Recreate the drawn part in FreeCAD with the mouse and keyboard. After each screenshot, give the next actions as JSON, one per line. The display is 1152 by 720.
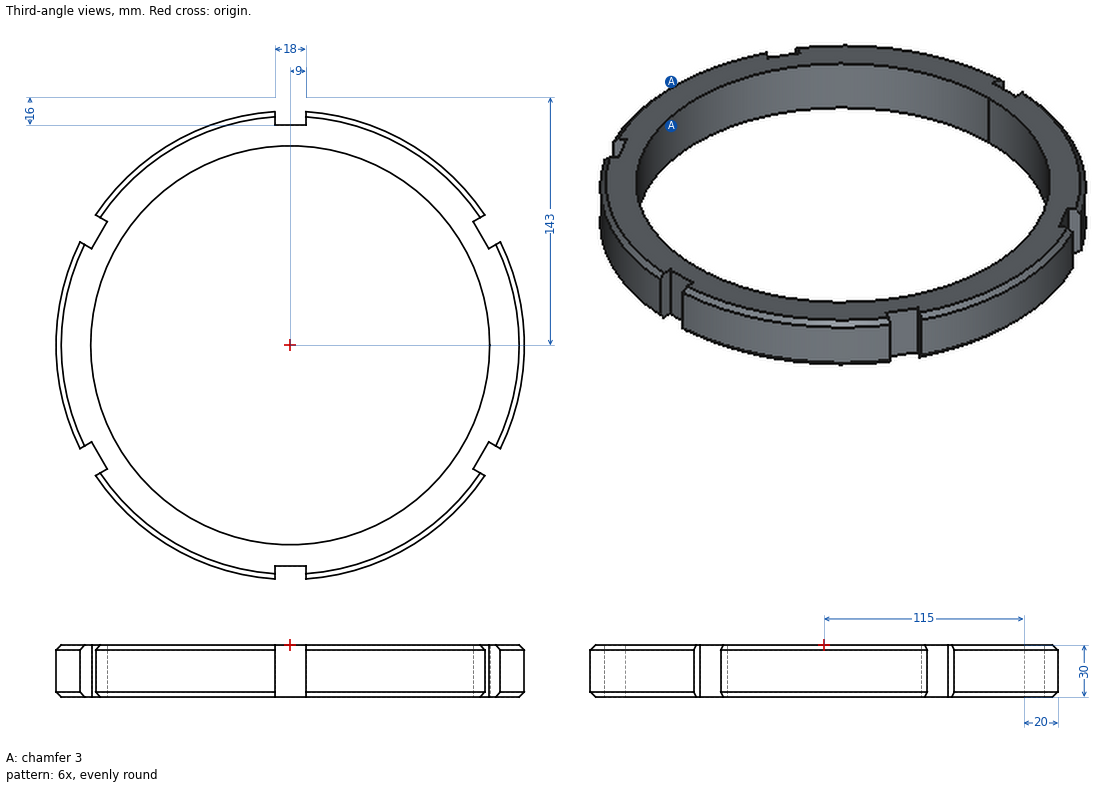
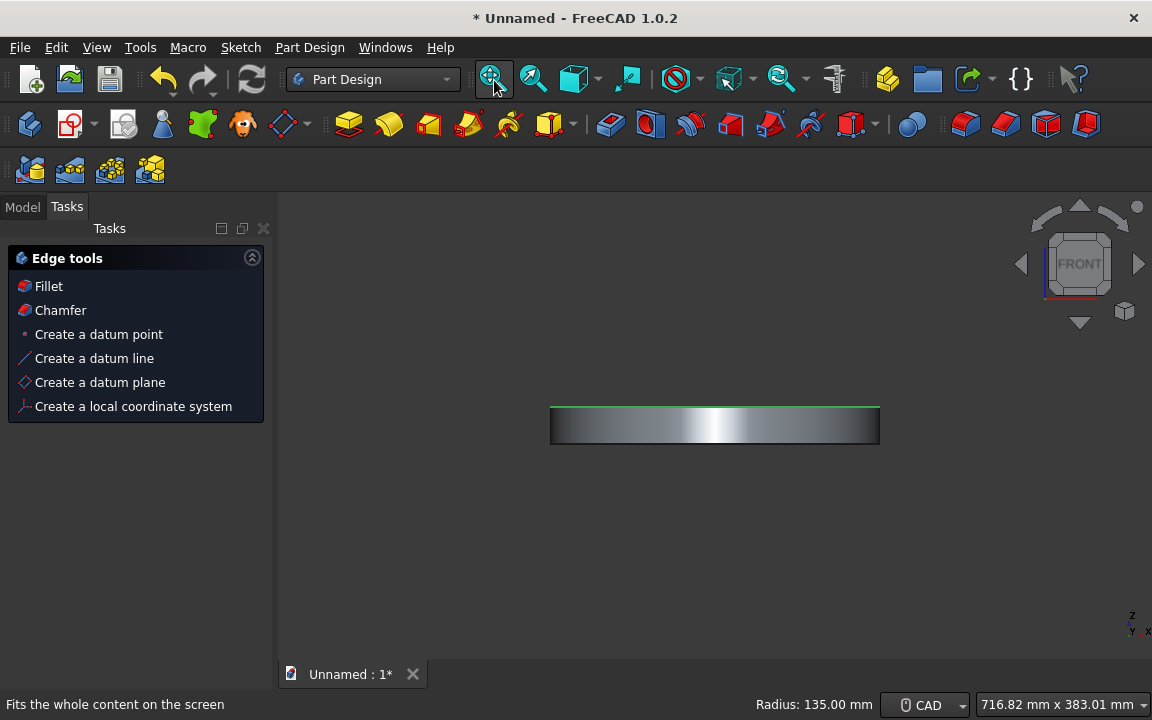
{"action": "left_click", "coordinate": [715, 443], "text": "ctrl"}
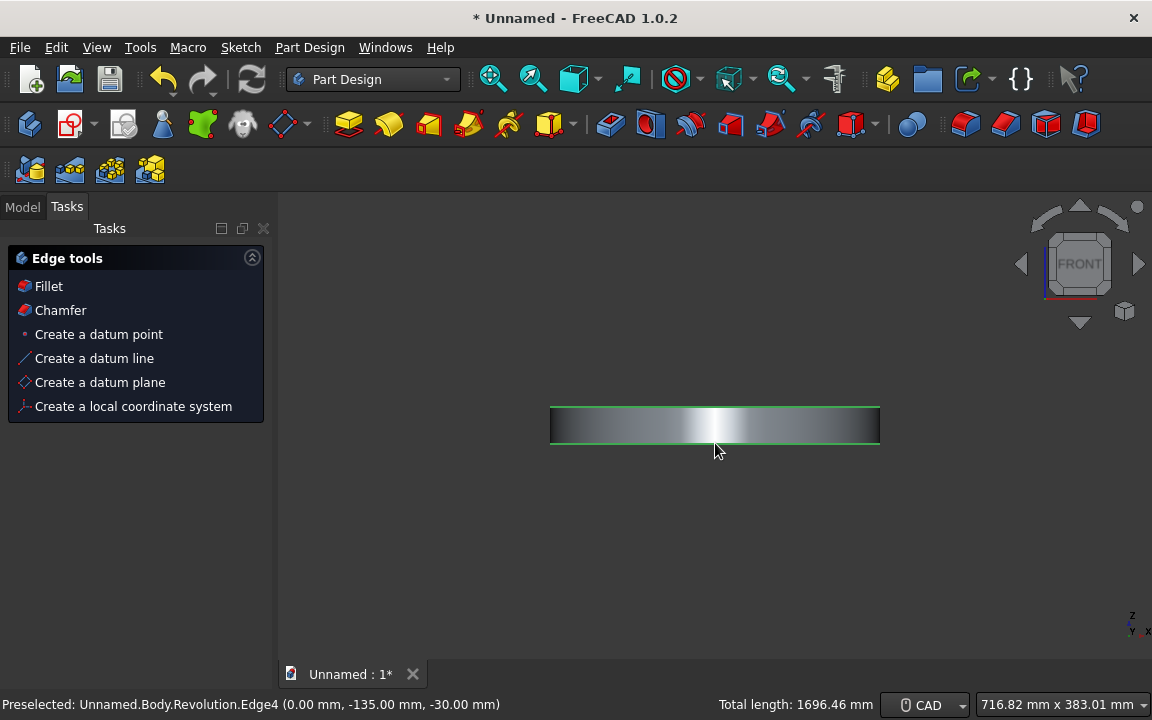
{"action": "left_click", "coordinate": [1006, 124]}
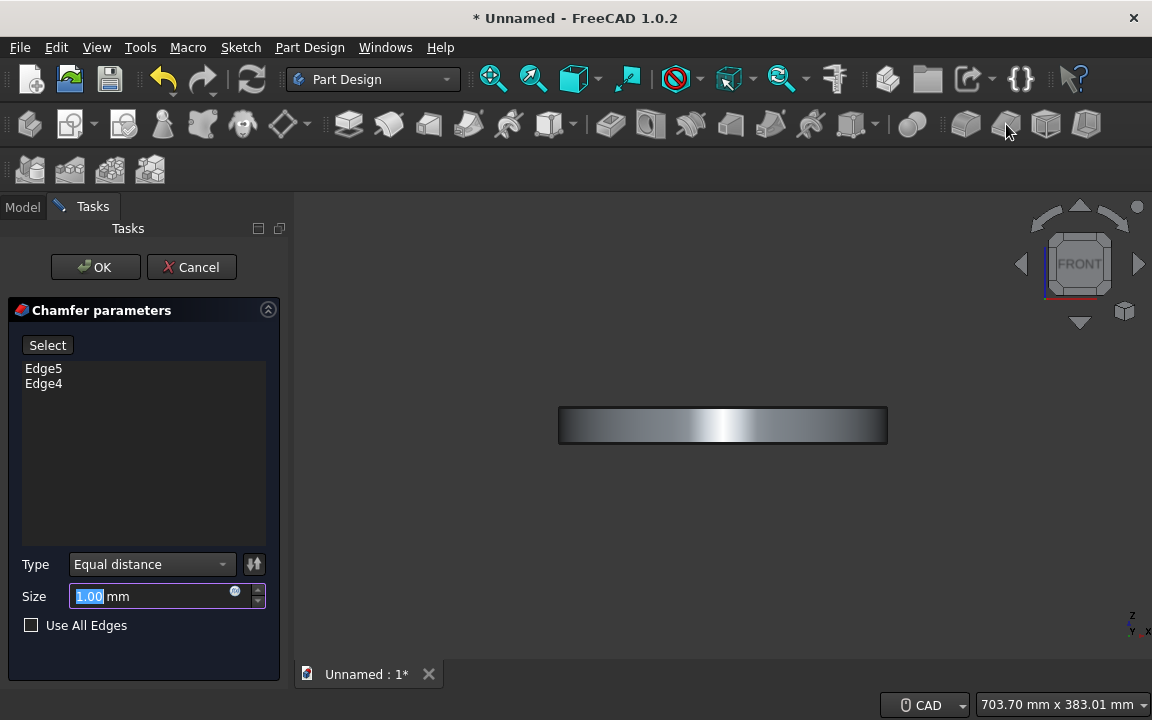
{"action": "type", "text": "3"}
{"action": "key", "text": "Tab"}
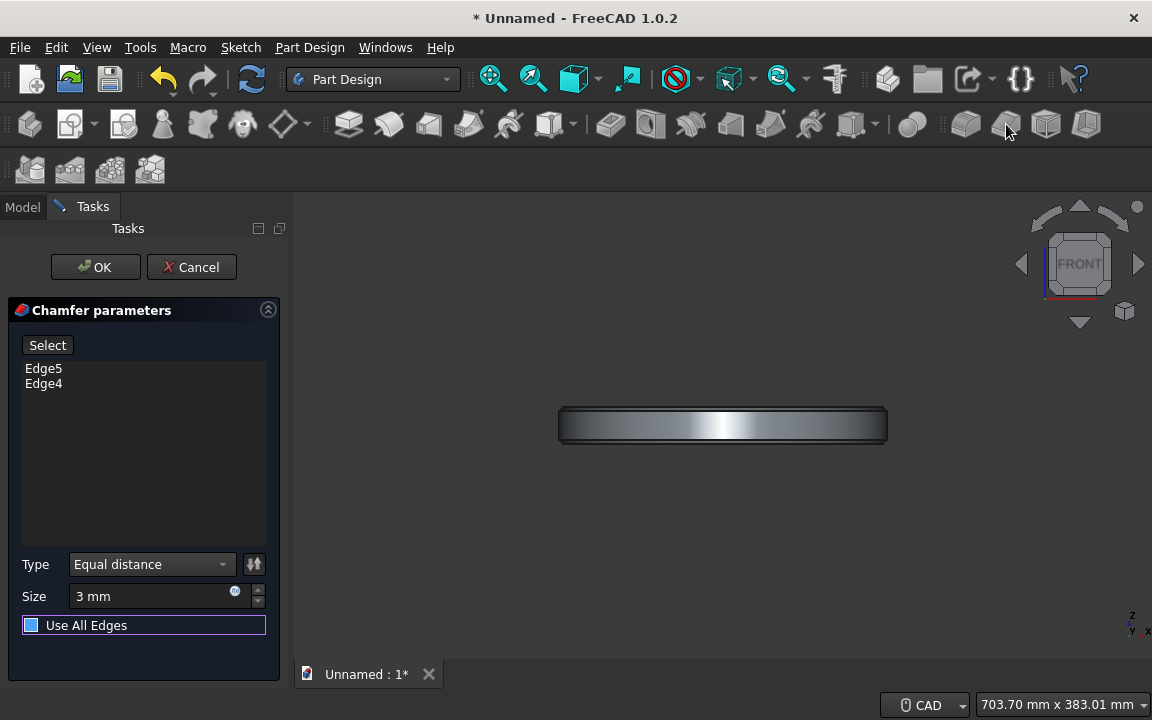
{"action": "left_click", "coordinate": [96, 267]}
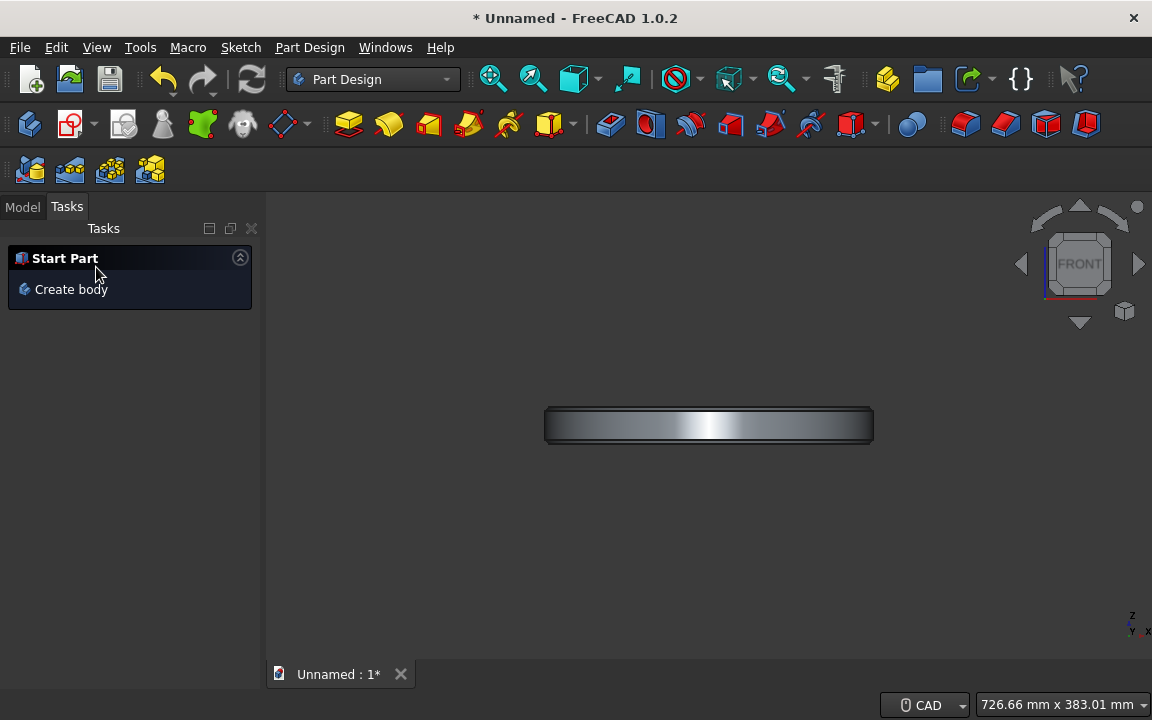
{"action": "left_click", "coordinate": [494, 80]}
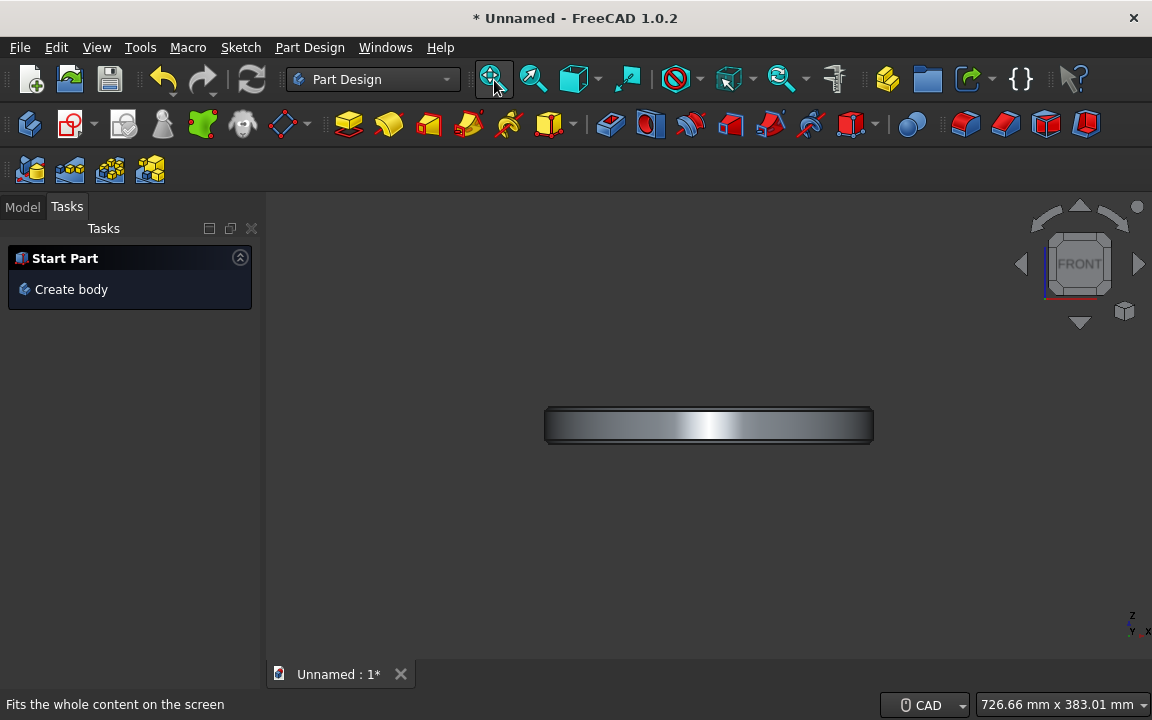
{"action": "key", "text": "0"}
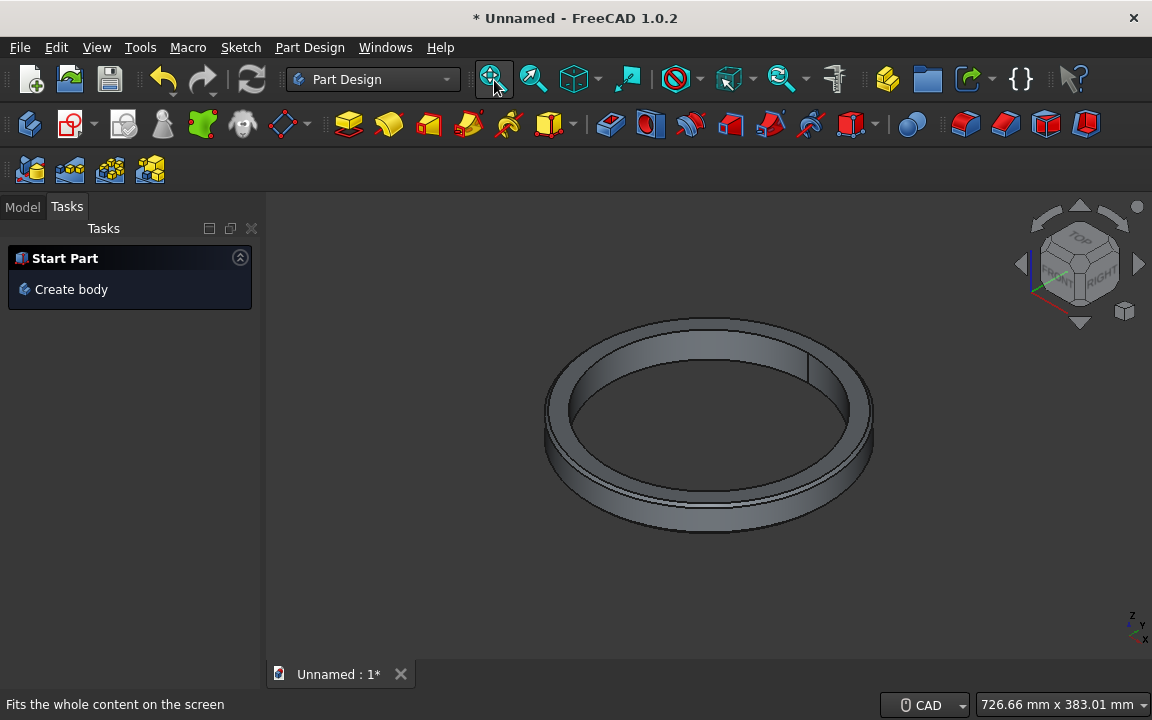
{"action": "left_click", "coordinate": [579, 447]}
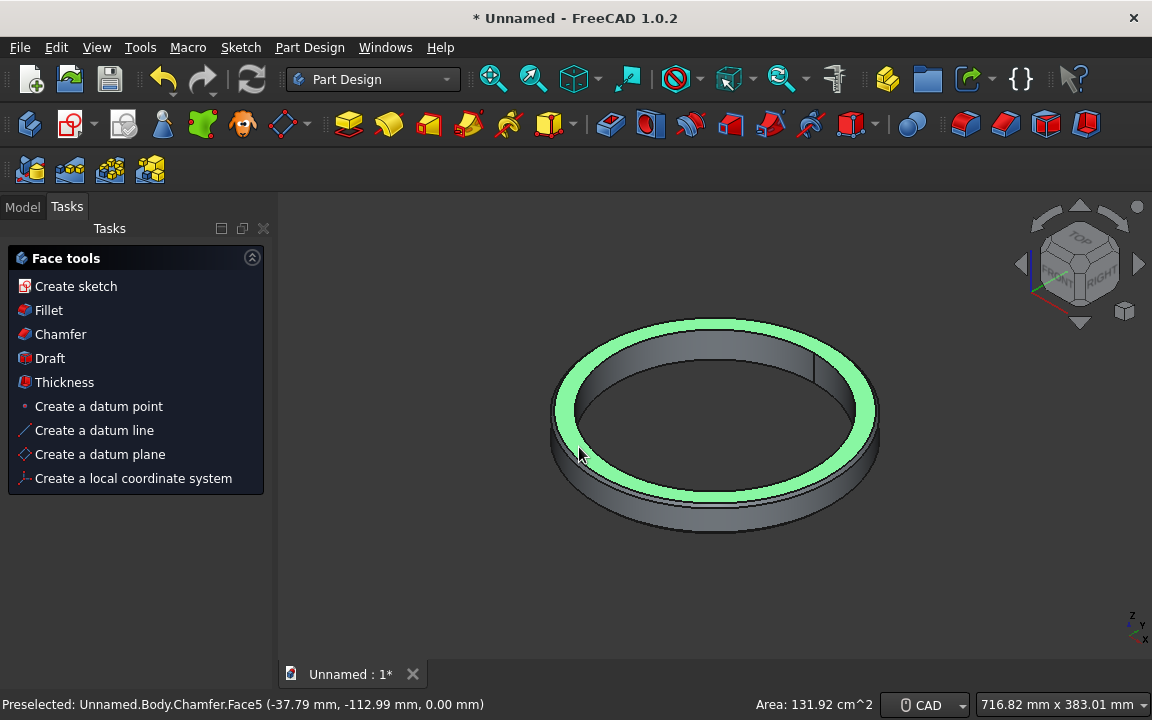
{"action": "left_click", "coordinate": [70, 124]}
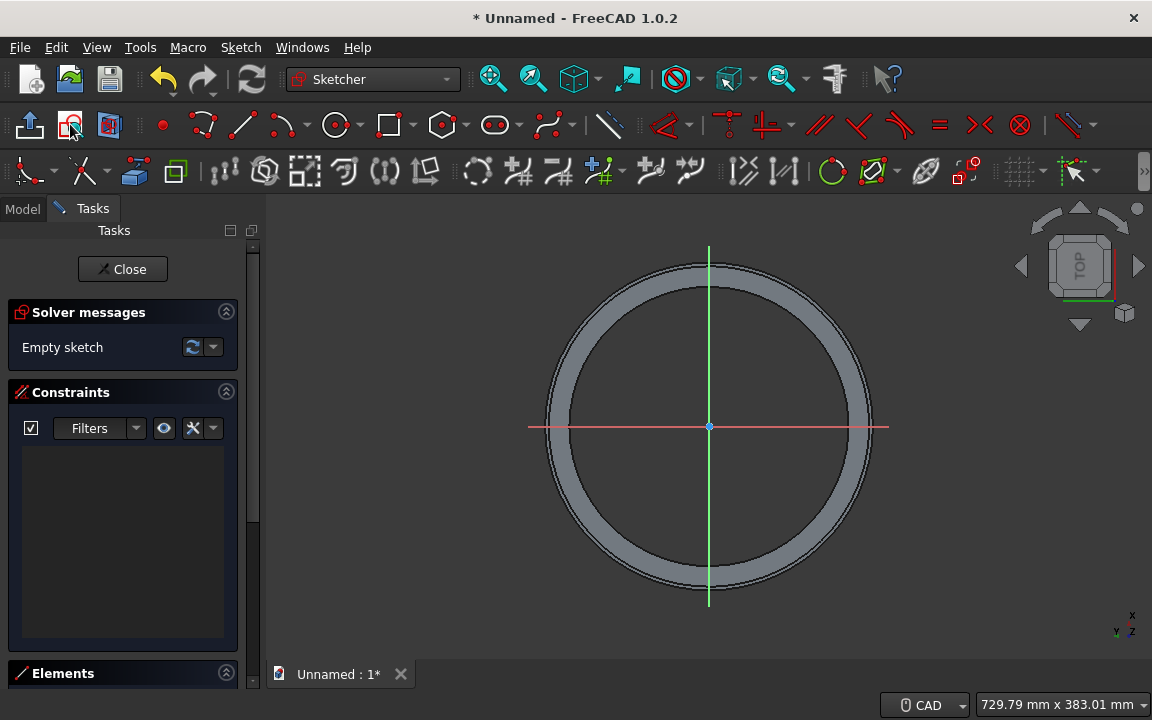
{"action": "scroll", "coordinate": [537, 426], "scroll_direction": "up", "scroll_amount": 13}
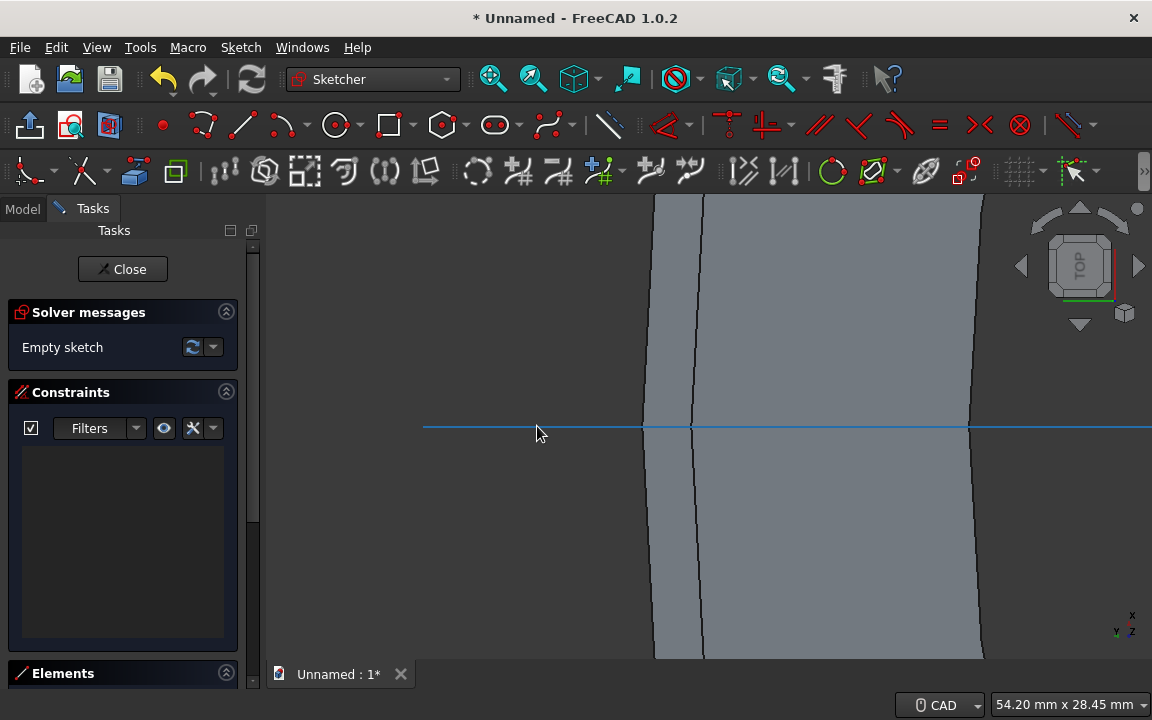
{"action": "left_click", "coordinate": [390, 126]}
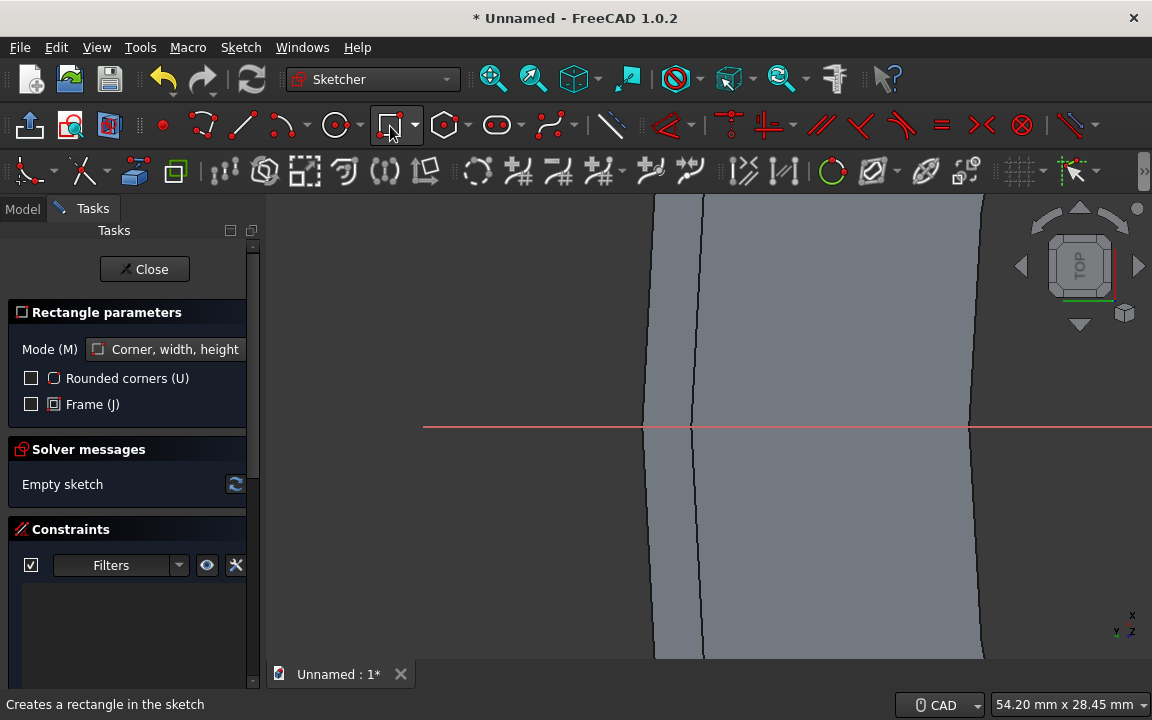
{"action": "left_click", "coordinate": [512, 279]}
{"action": "left_click", "coordinate": [773, 574]}
{"action": "key", "text": "Escape"}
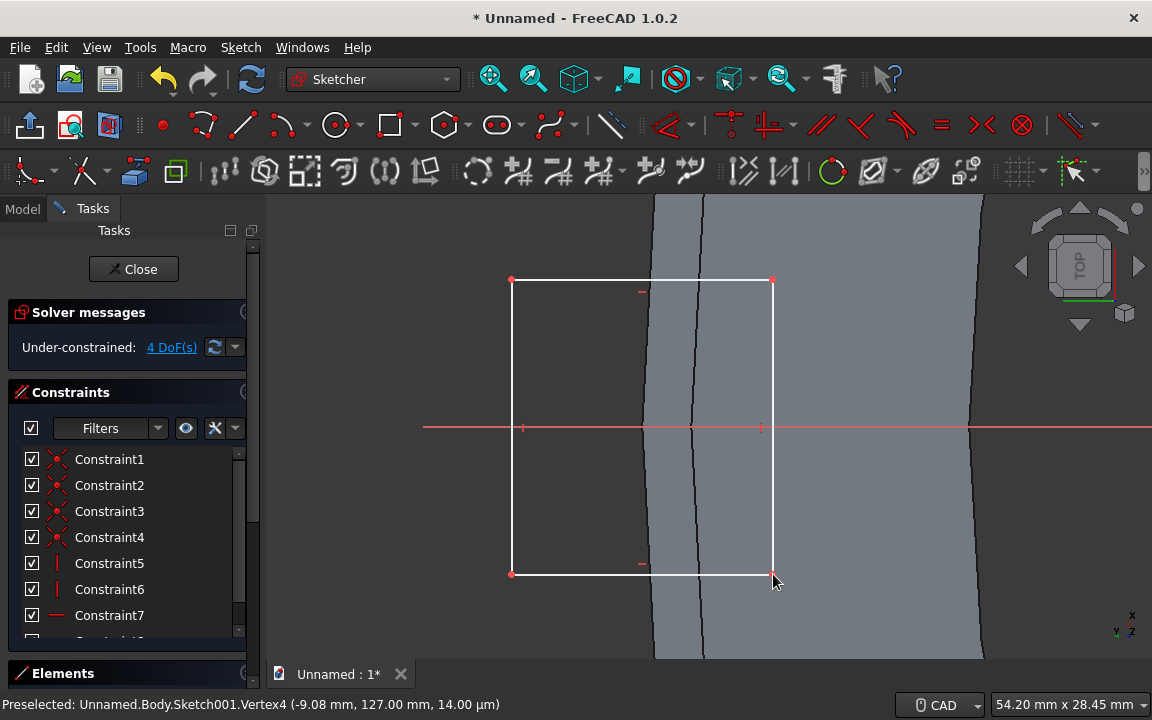
{"action": "left_click", "coordinate": [666, 126]}